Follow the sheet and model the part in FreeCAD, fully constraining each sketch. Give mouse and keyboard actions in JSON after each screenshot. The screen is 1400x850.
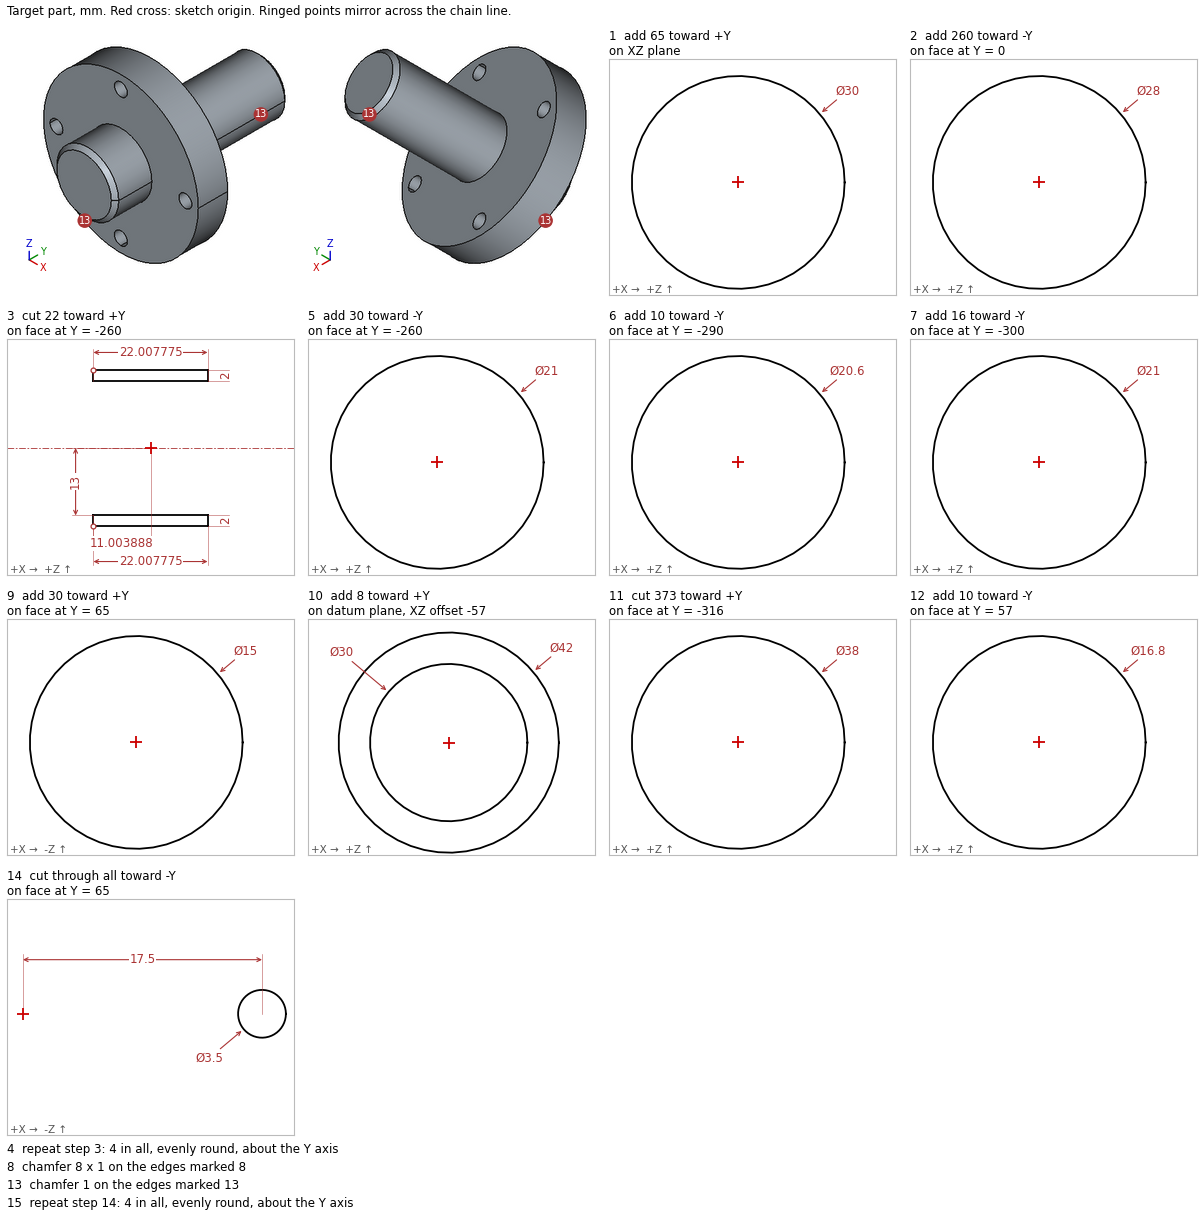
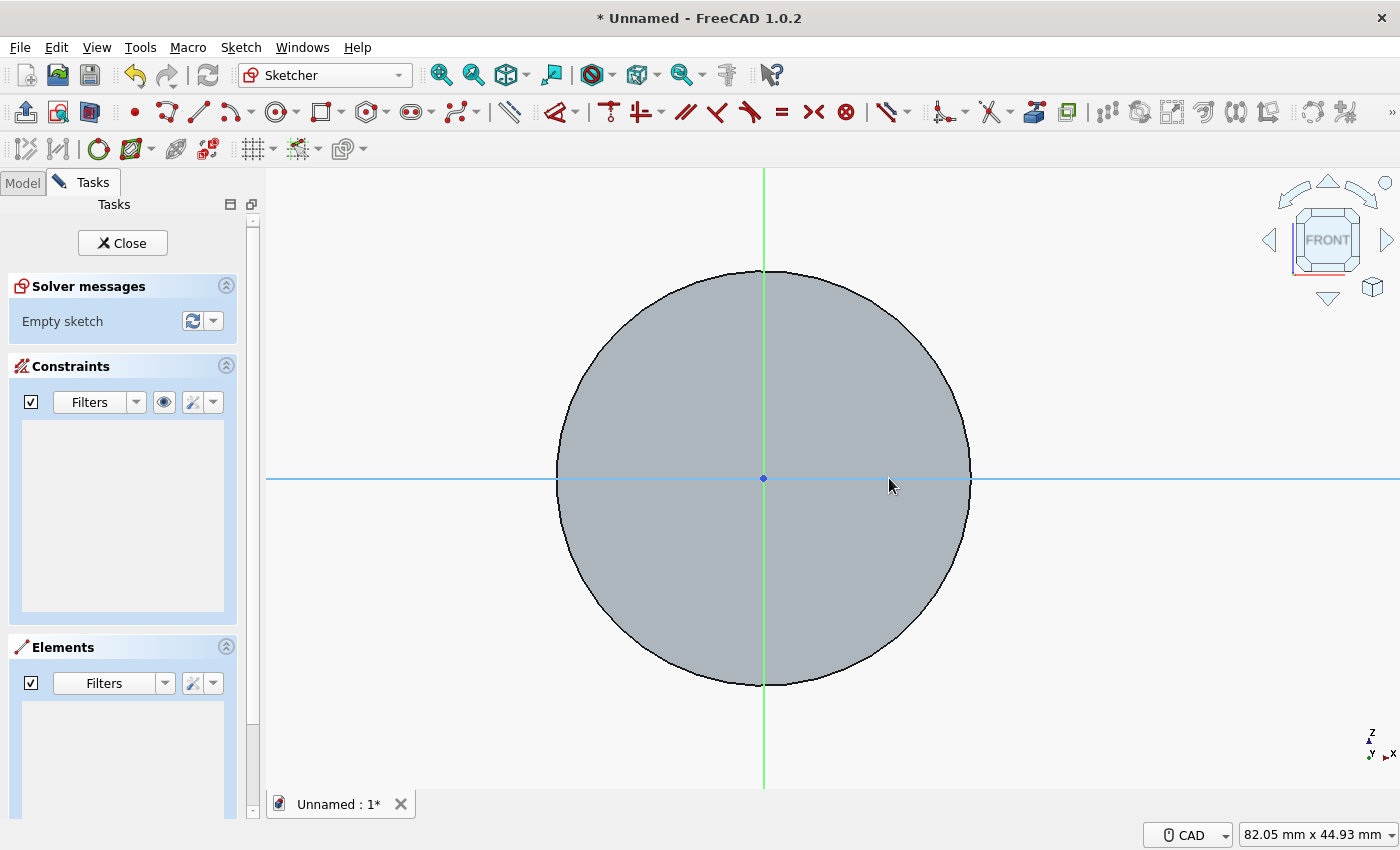
{"action": "left_click", "coordinate": [276, 112]}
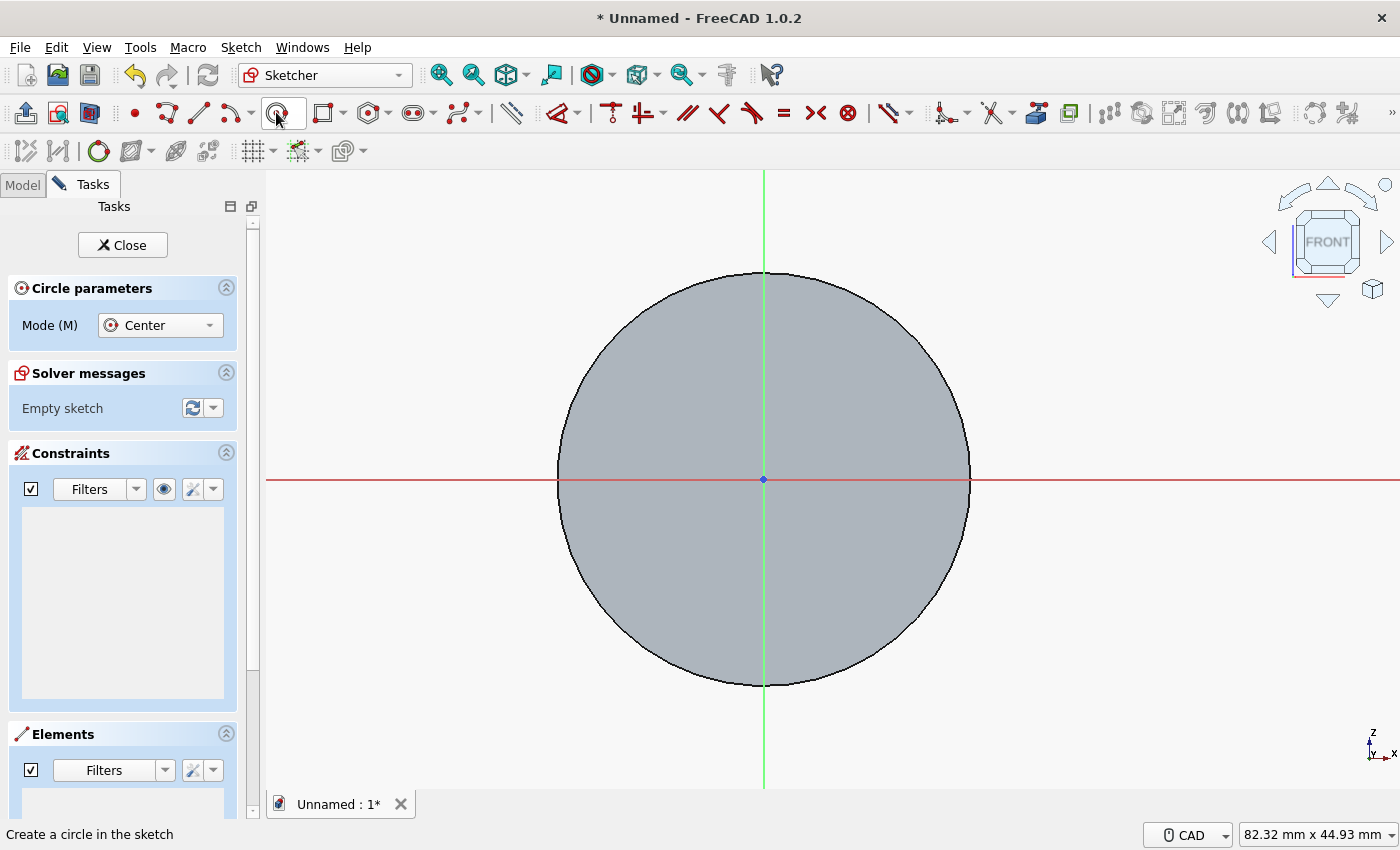
{"action": "left_click", "coordinate": [764, 480]}
{"action": "mouse_move", "coordinate": [900, 343]}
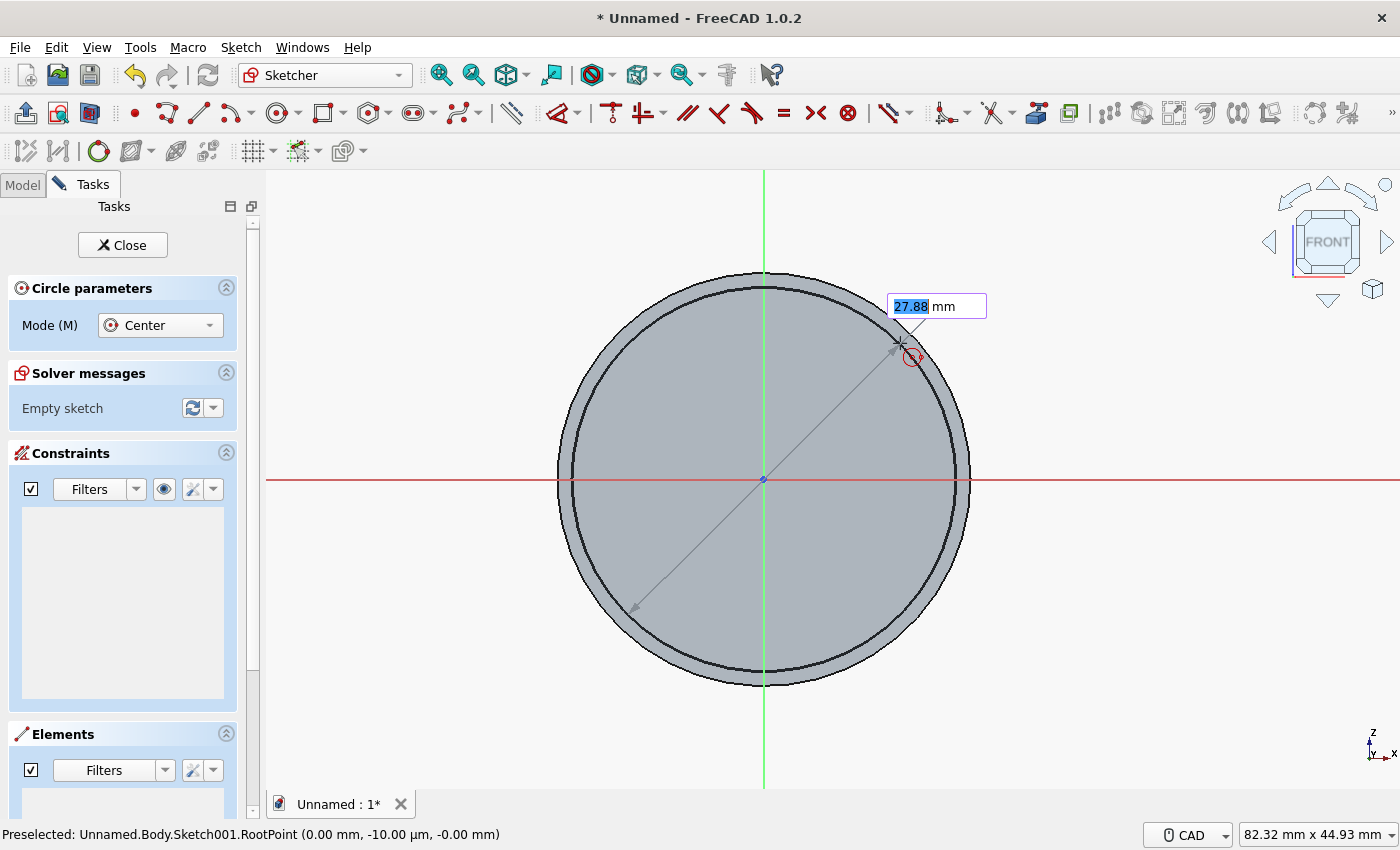
{"action": "type", "text": "28"}
{"action": "key", "text": "Return"}
{"action": "key", "text": "Escape"}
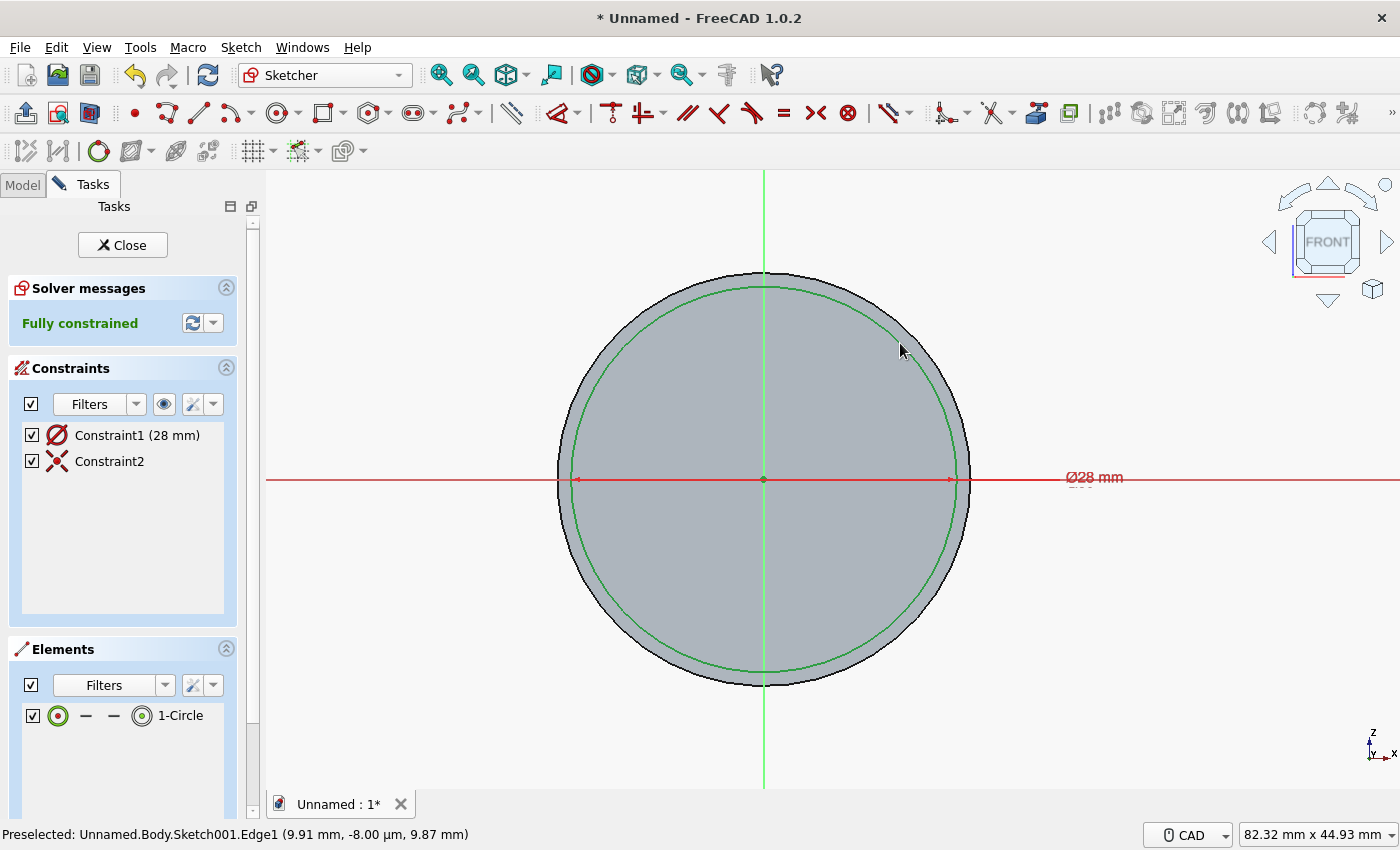
{"action": "left_click", "coordinate": [123, 245]}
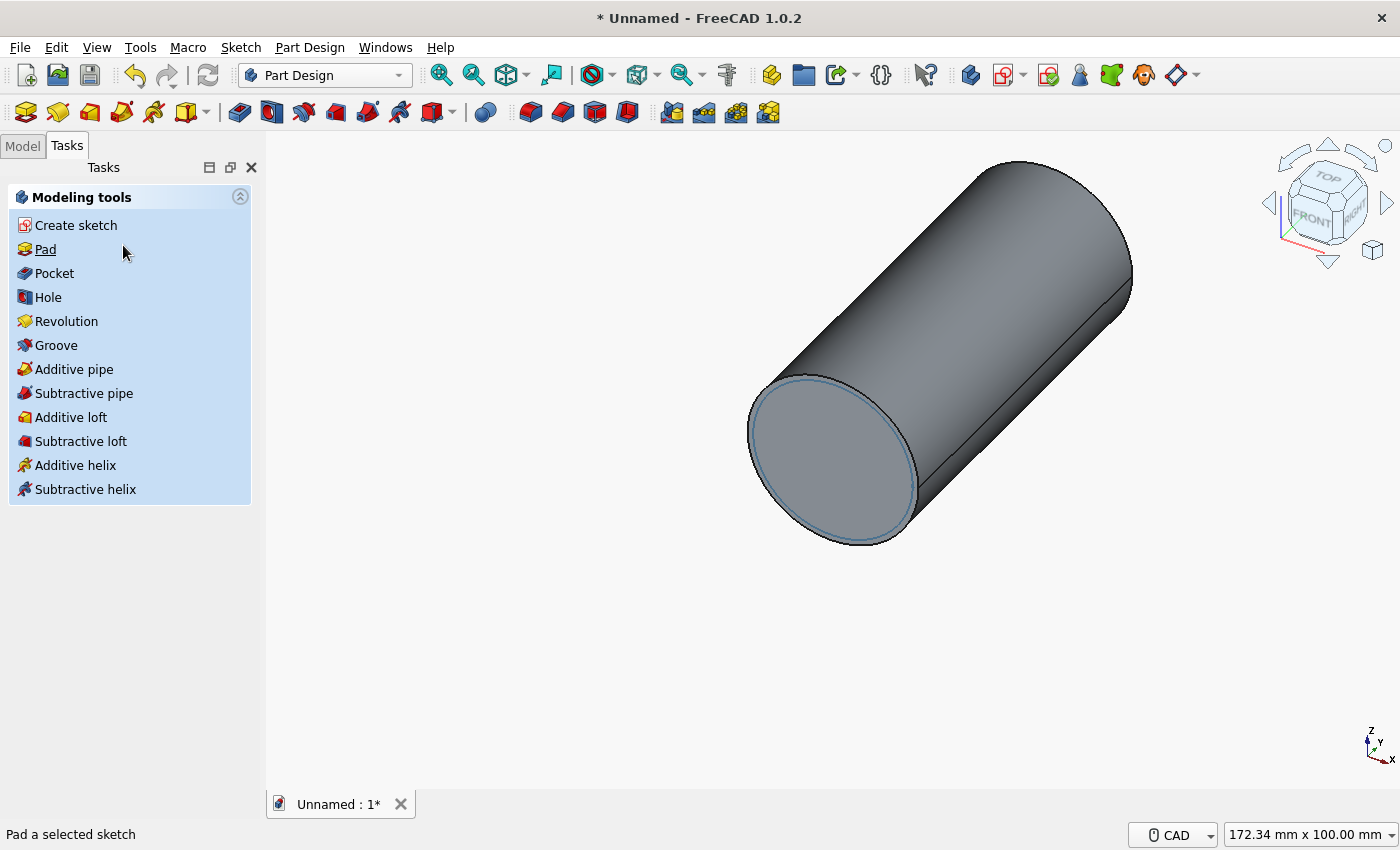
{"action": "left_click", "coordinate": [26, 112]}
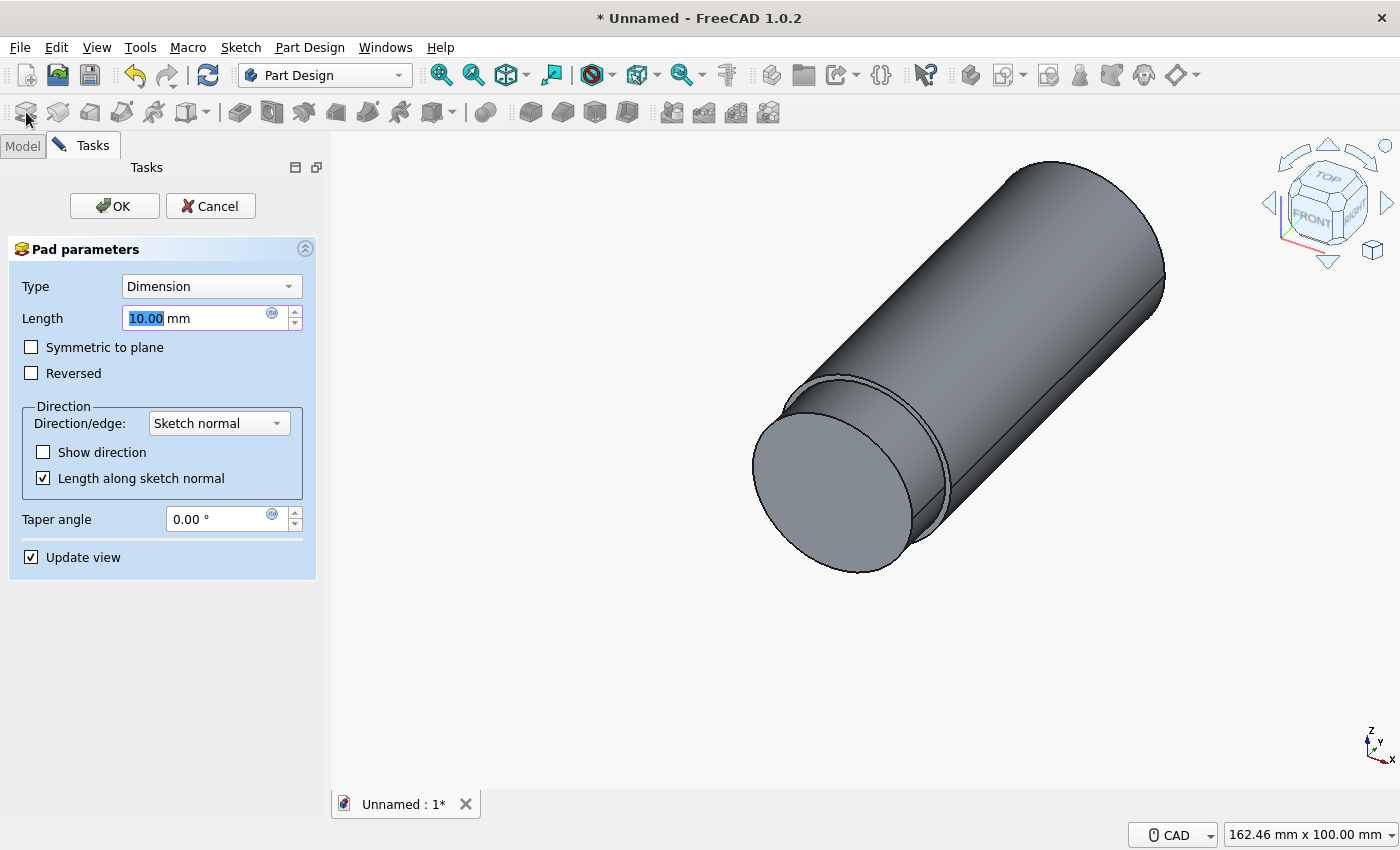
{"action": "type", "text": "260"}
{"action": "key", "text": "Tab"}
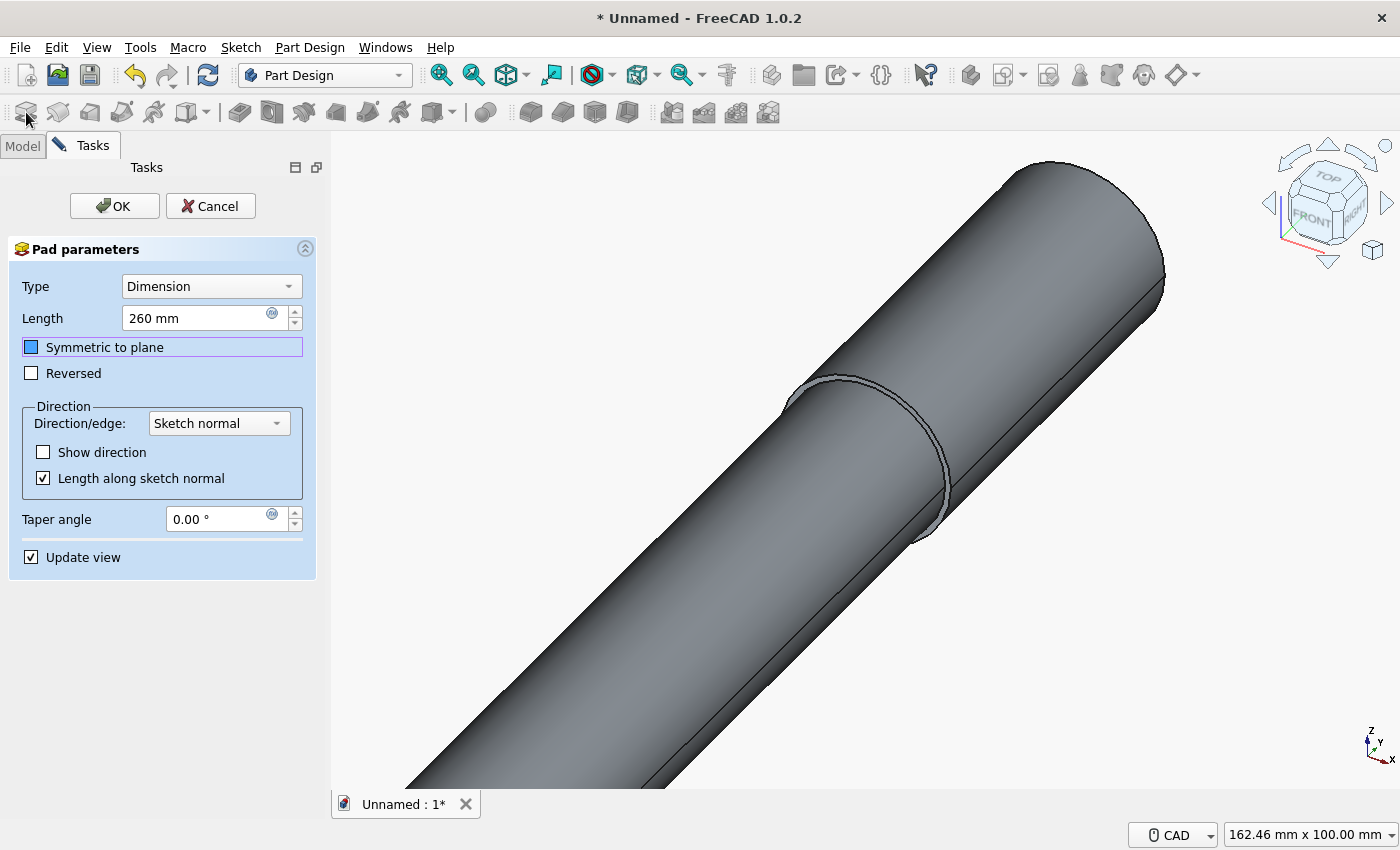
{"action": "left_click", "coordinate": [115, 206]}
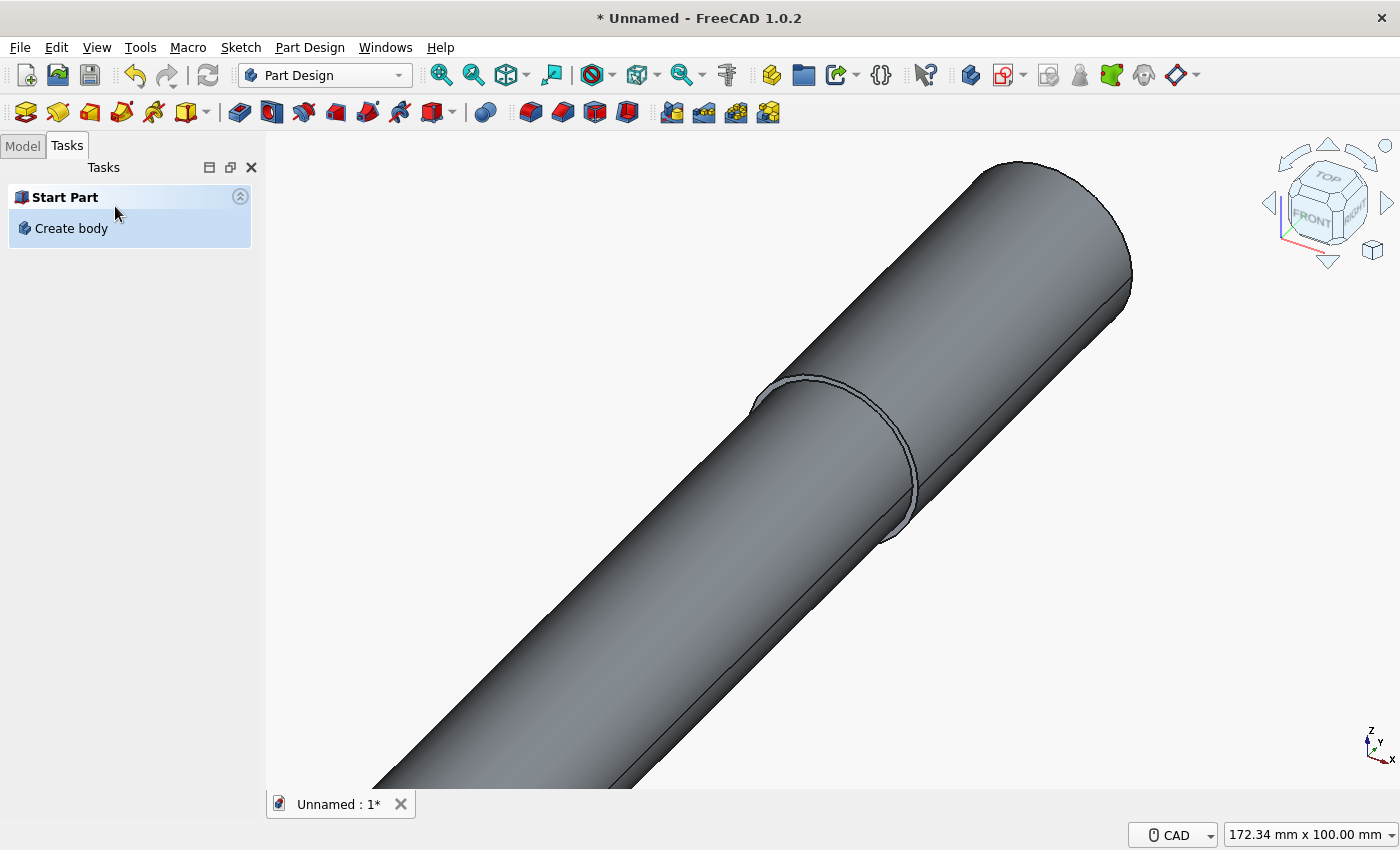
{"action": "left_click", "coordinate": [442, 76]}